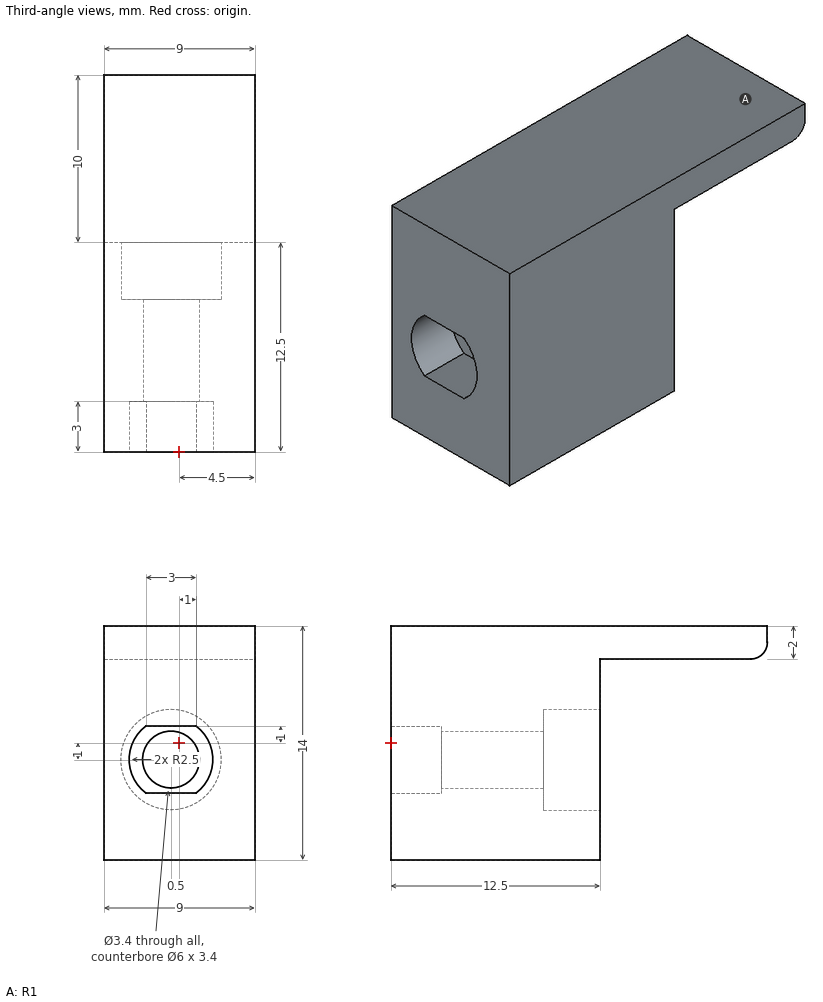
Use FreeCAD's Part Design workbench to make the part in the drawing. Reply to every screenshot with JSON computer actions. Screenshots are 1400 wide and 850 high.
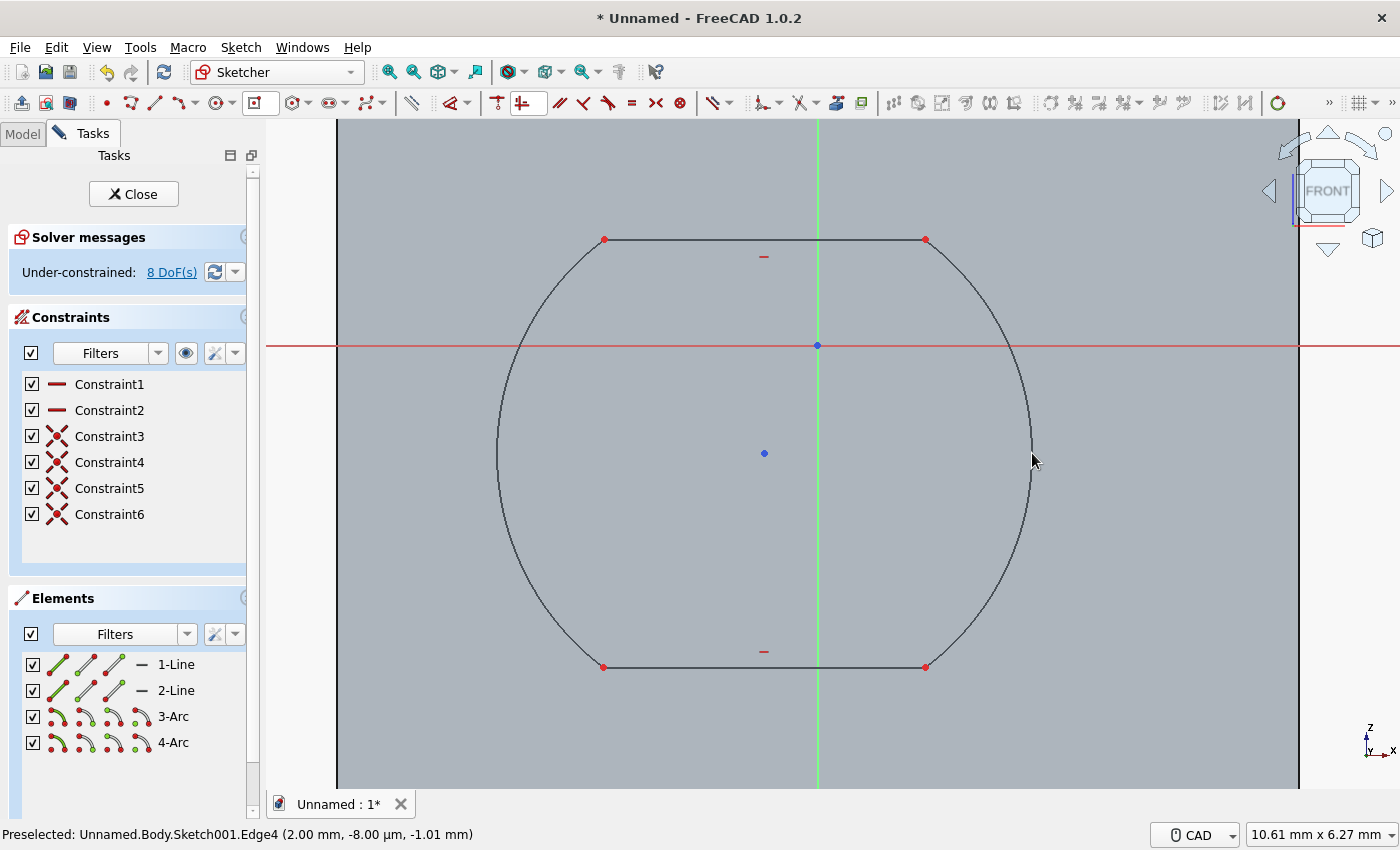
{"action": "scroll", "coordinate": [515, 357], "scroll_direction": "up", "scroll_amount": 2}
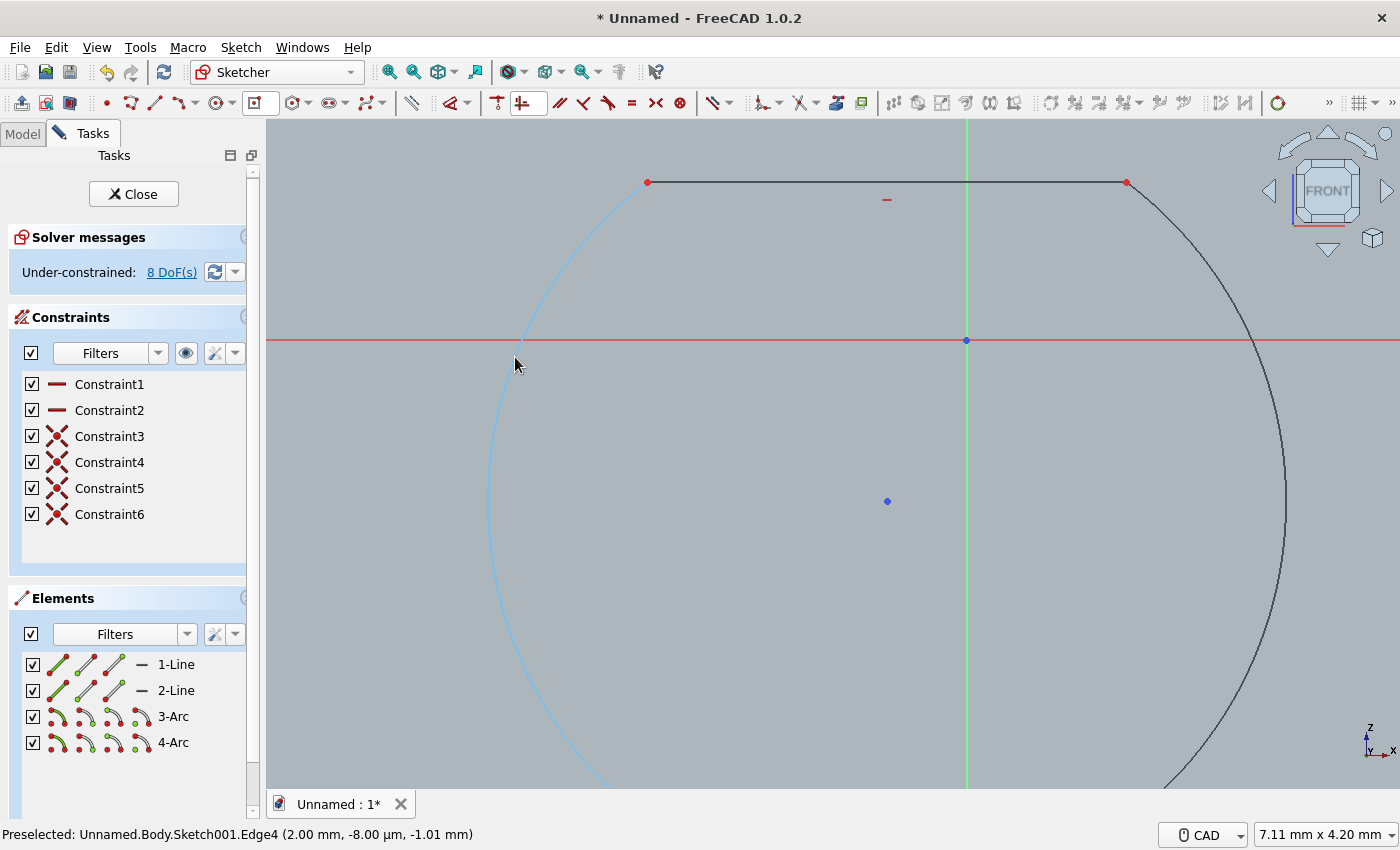
{"action": "left_click", "coordinate": [515, 357]}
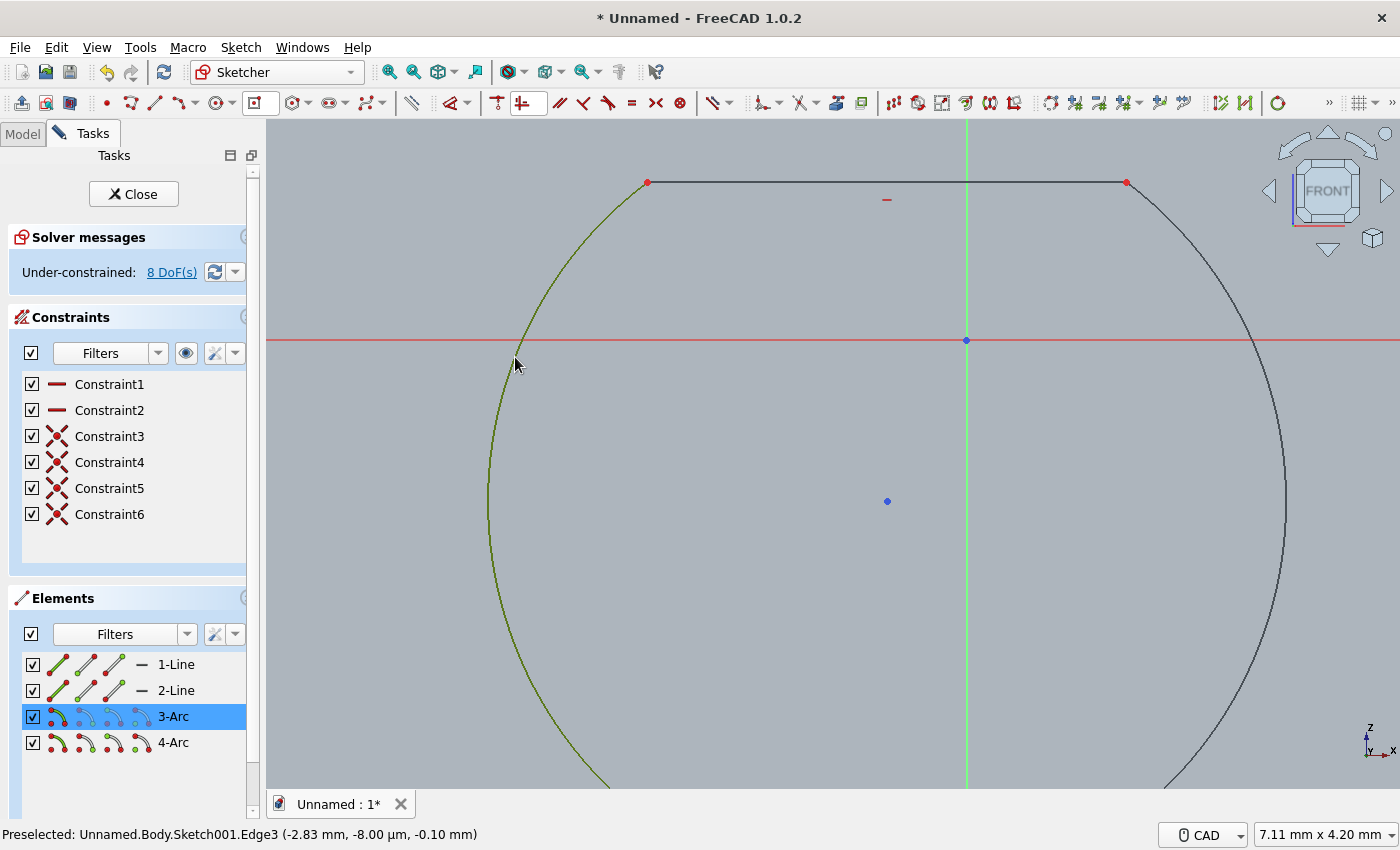
{"action": "left_click", "coordinate": [1226, 712]}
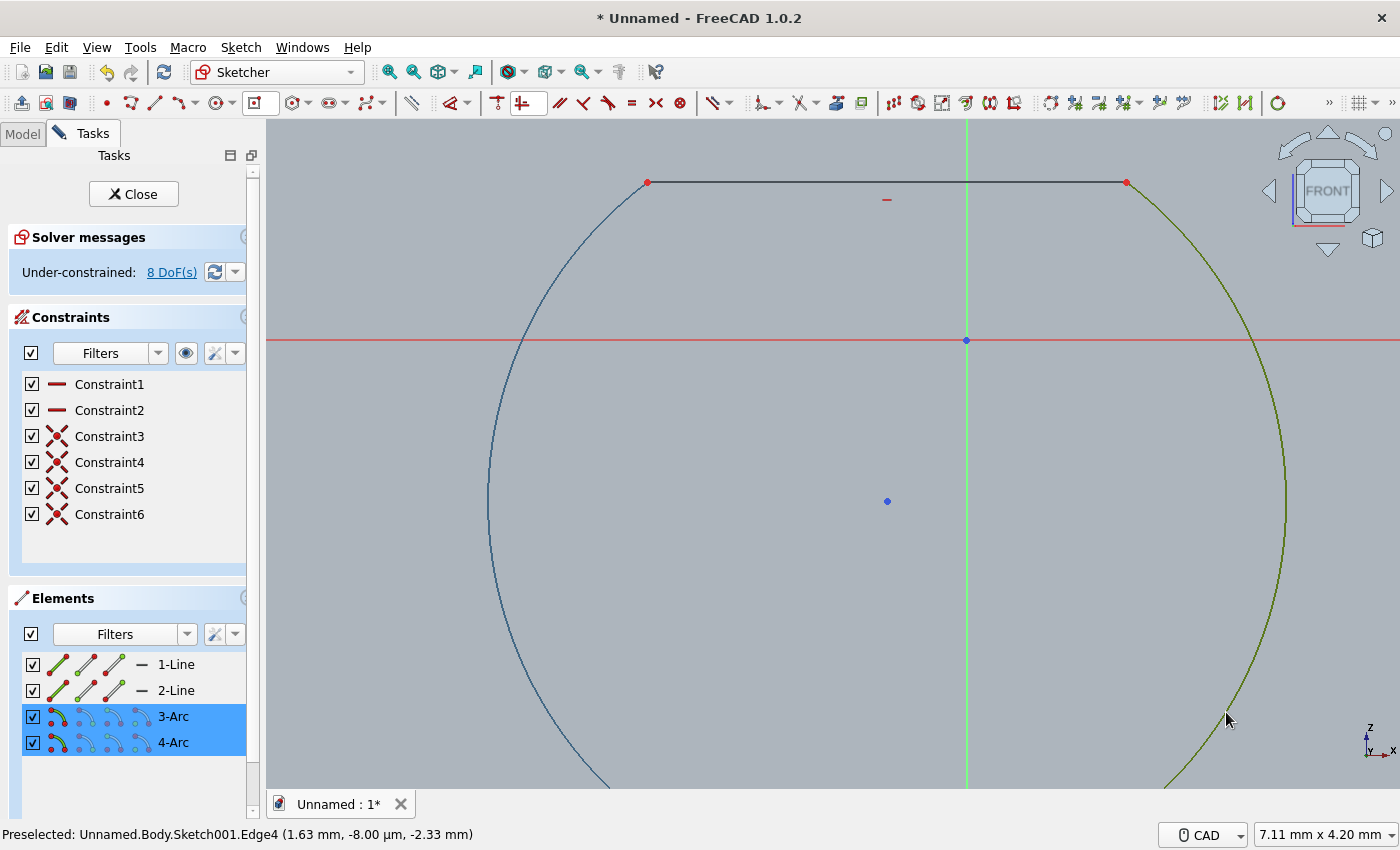
{"action": "key", "text": "c"}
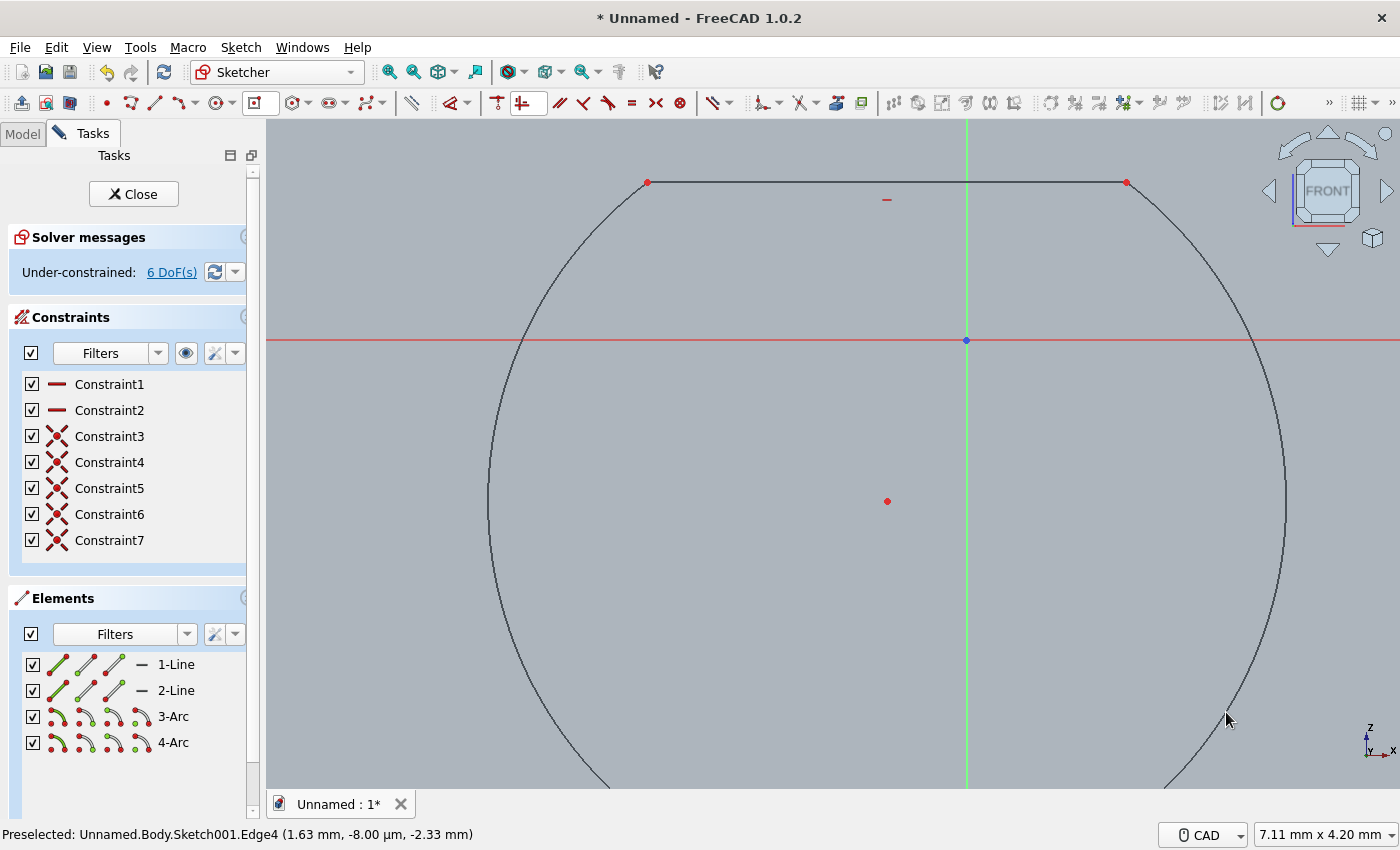
{"action": "left_click", "coordinate": [515, 357]}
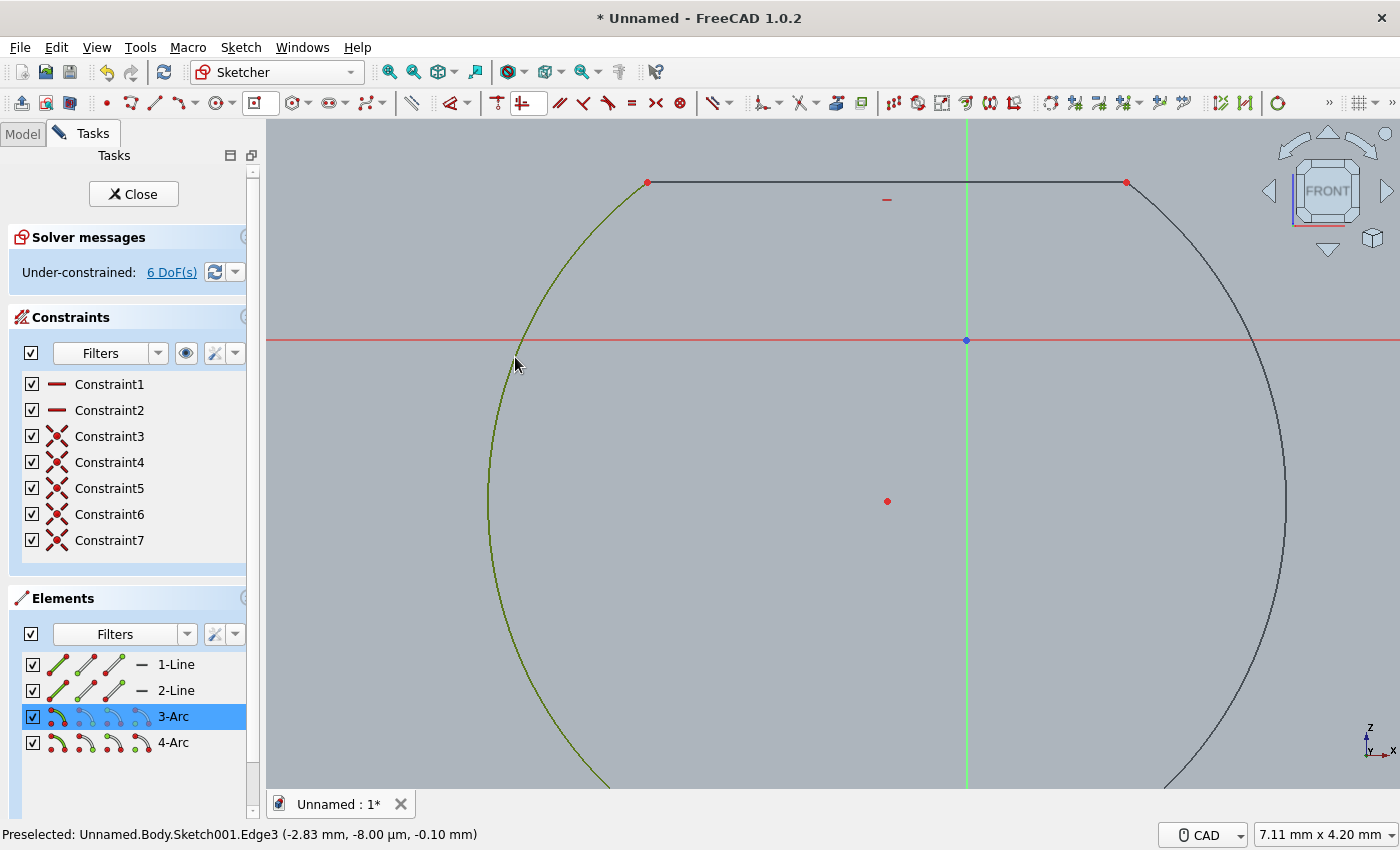
{"action": "left_click", "coordinate": [1226, 712]}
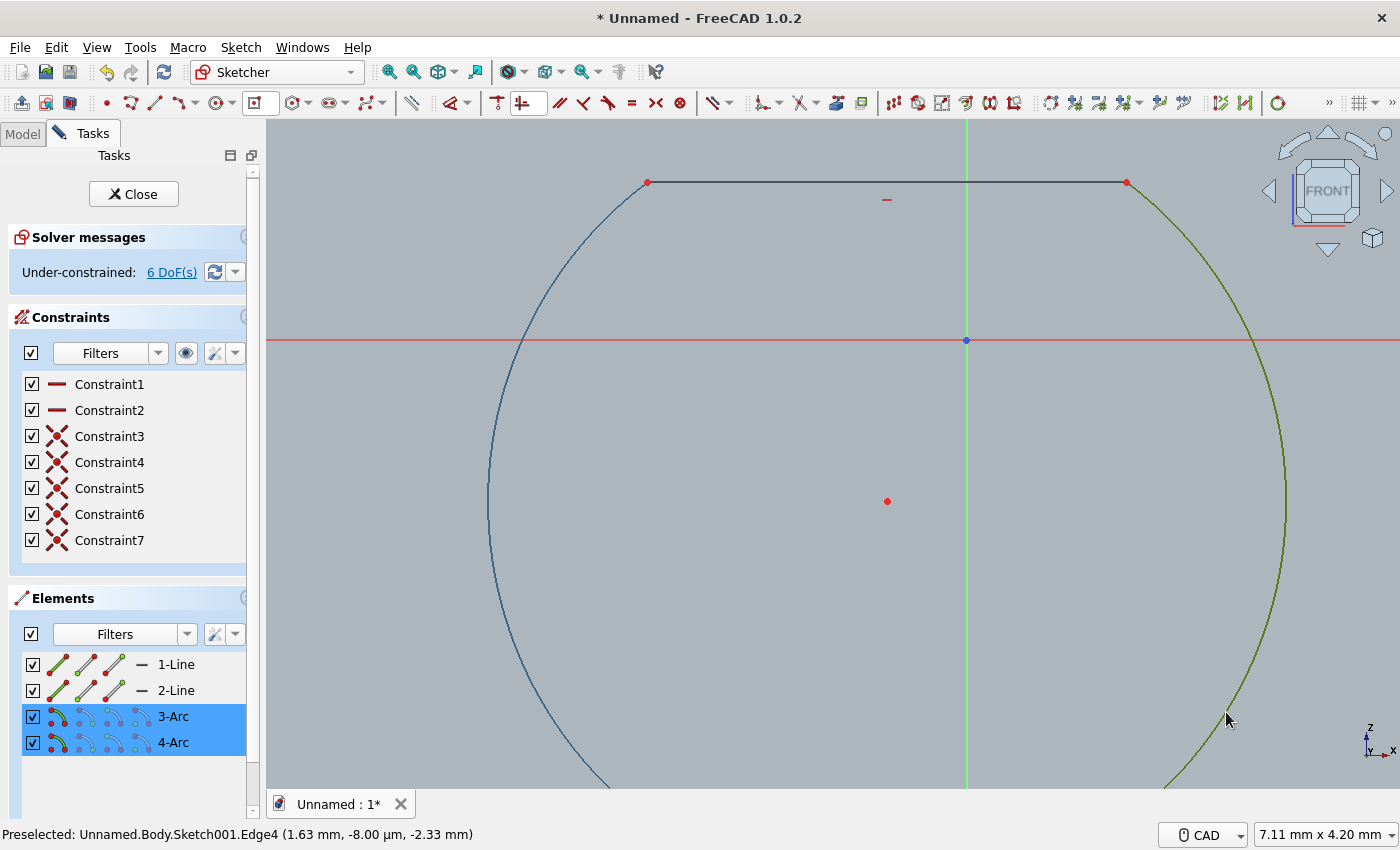
{"action": "key", "text": "e"}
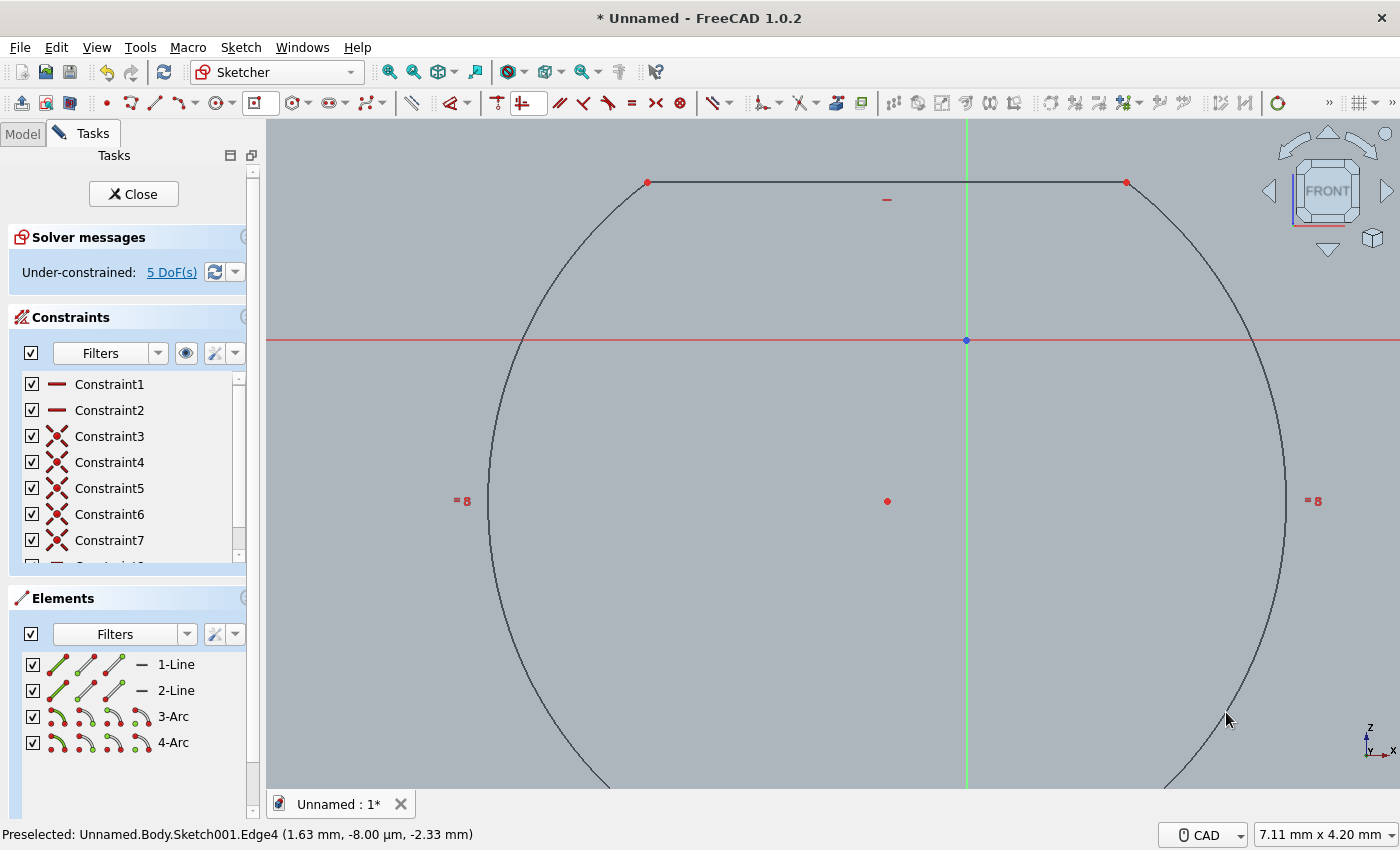
{"action": "key", "text": "d"}